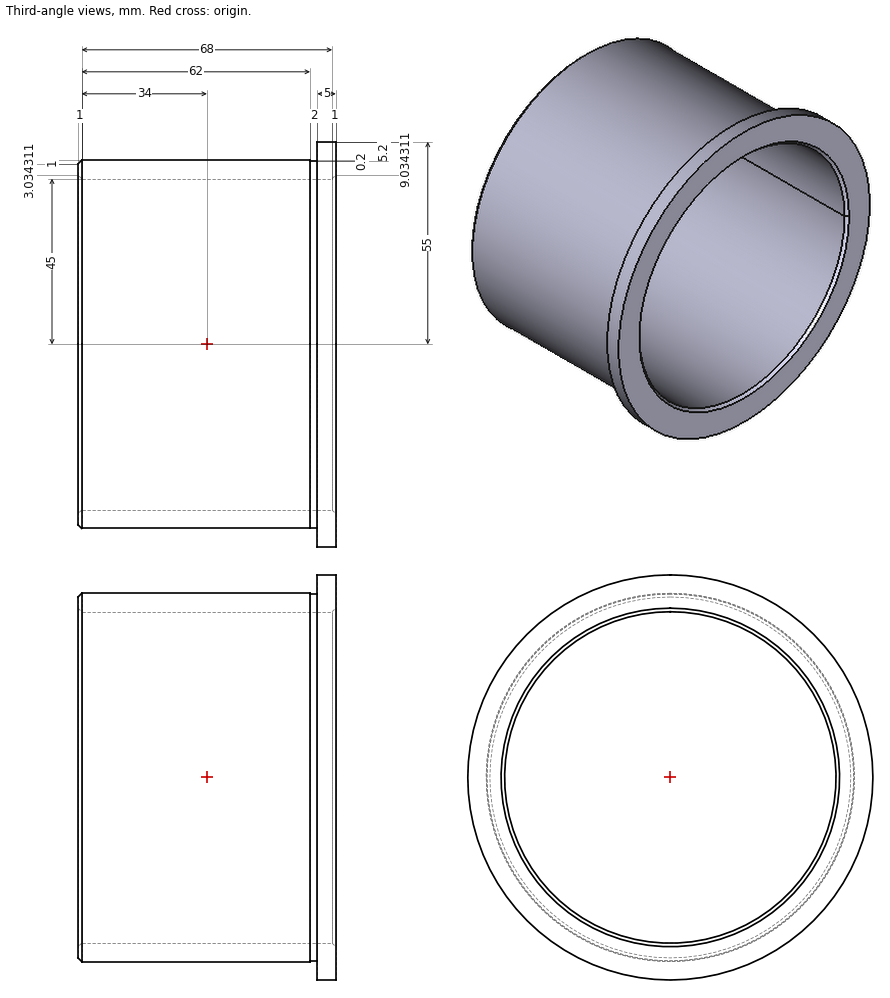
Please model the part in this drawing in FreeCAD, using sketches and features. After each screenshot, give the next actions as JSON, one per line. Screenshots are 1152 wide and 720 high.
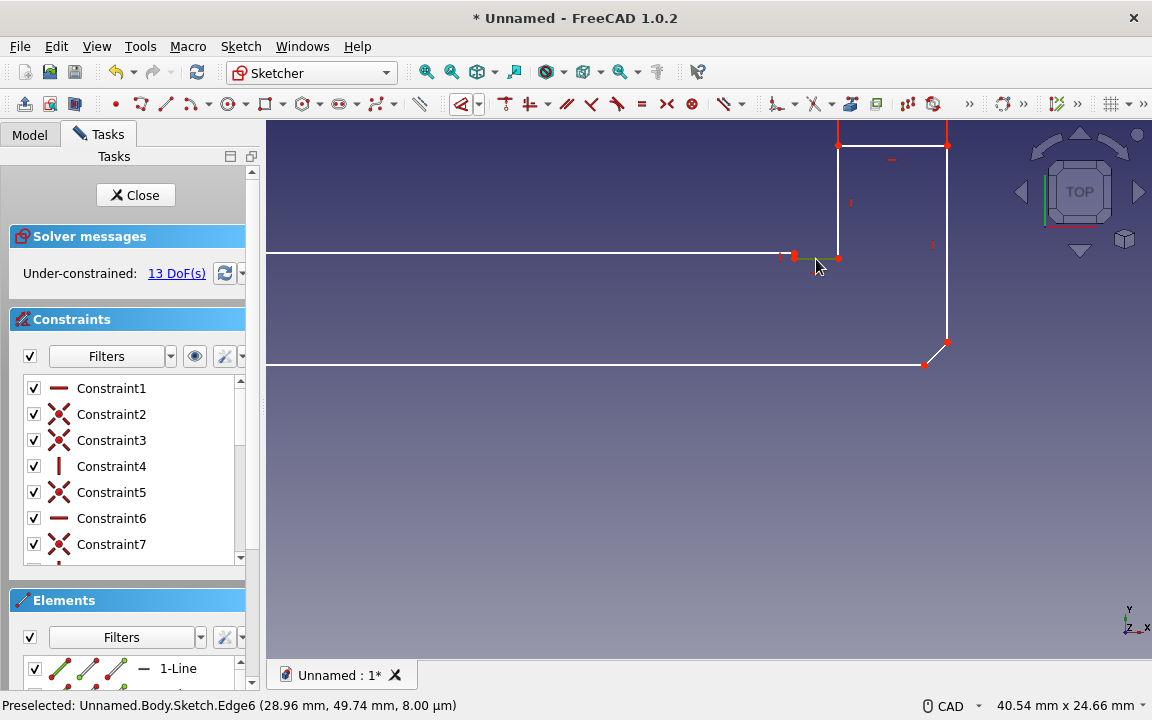
{"action": "key", "text": "l"}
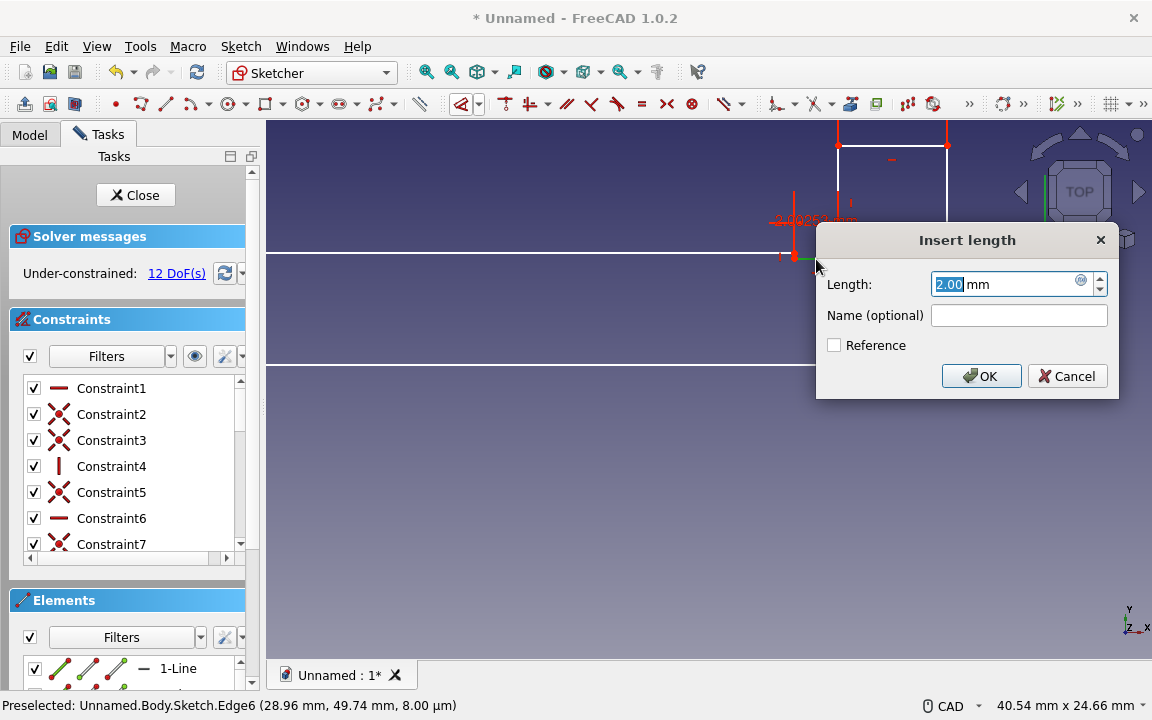
{"action": "type", "text": "2"}
{"action": "key", "text": "Return"}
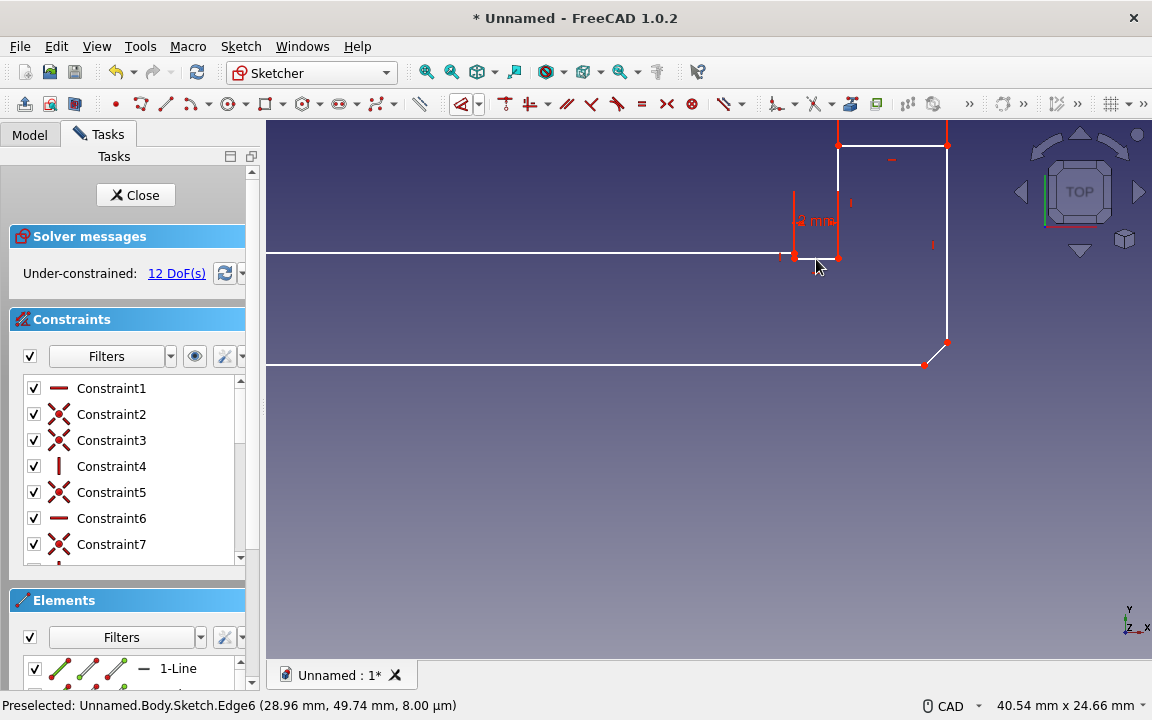
{"action": "left_click", "coordinate": [480, 365]}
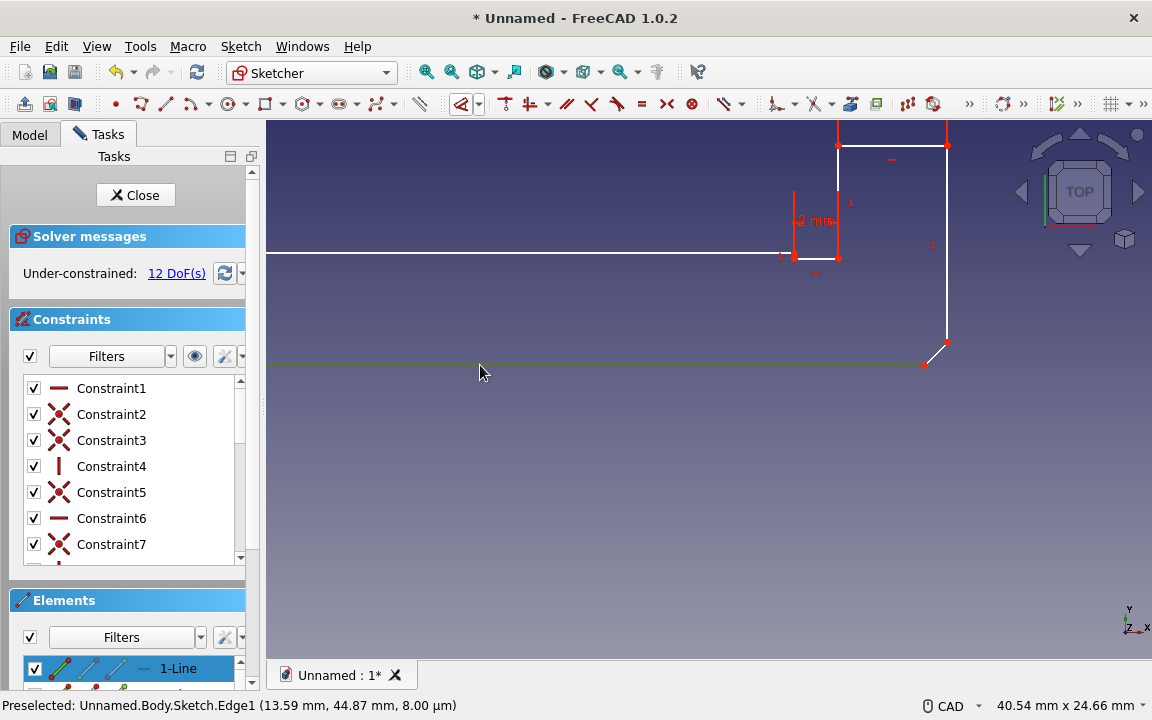
{"action": "key", "text": "l"}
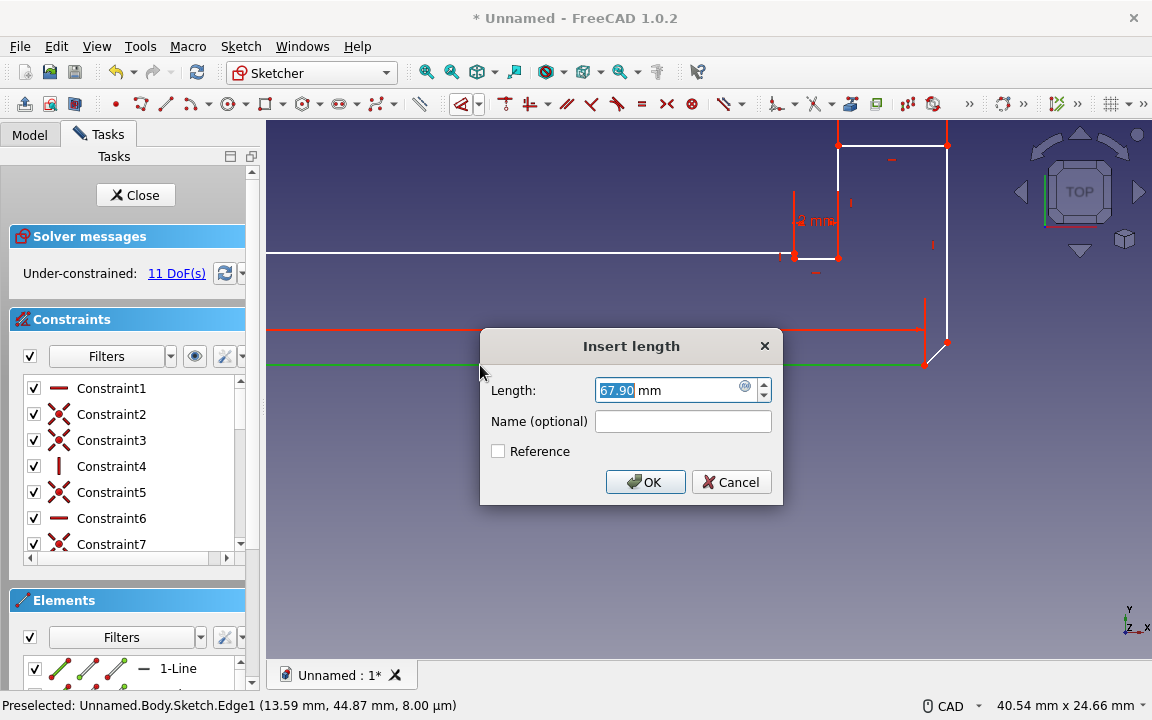
{"action": "type", "text": "68"}
{"action": "key", "text": "Return"}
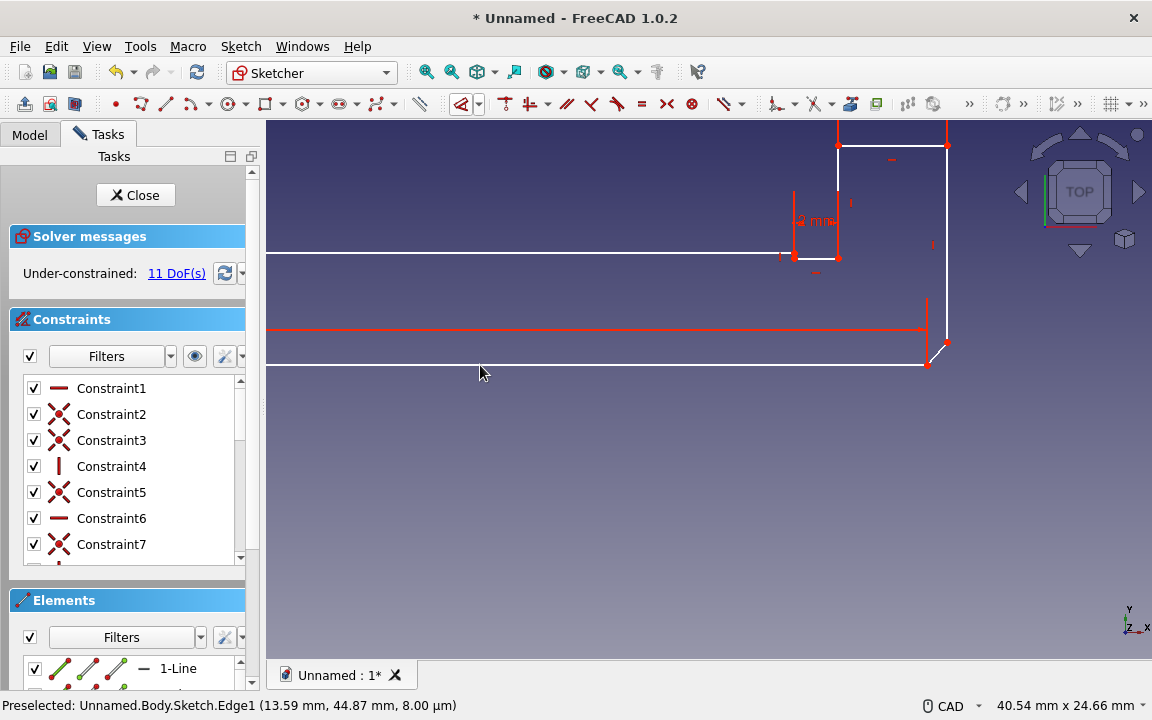
{"action": "left_click", "coordinate": [388, 253]}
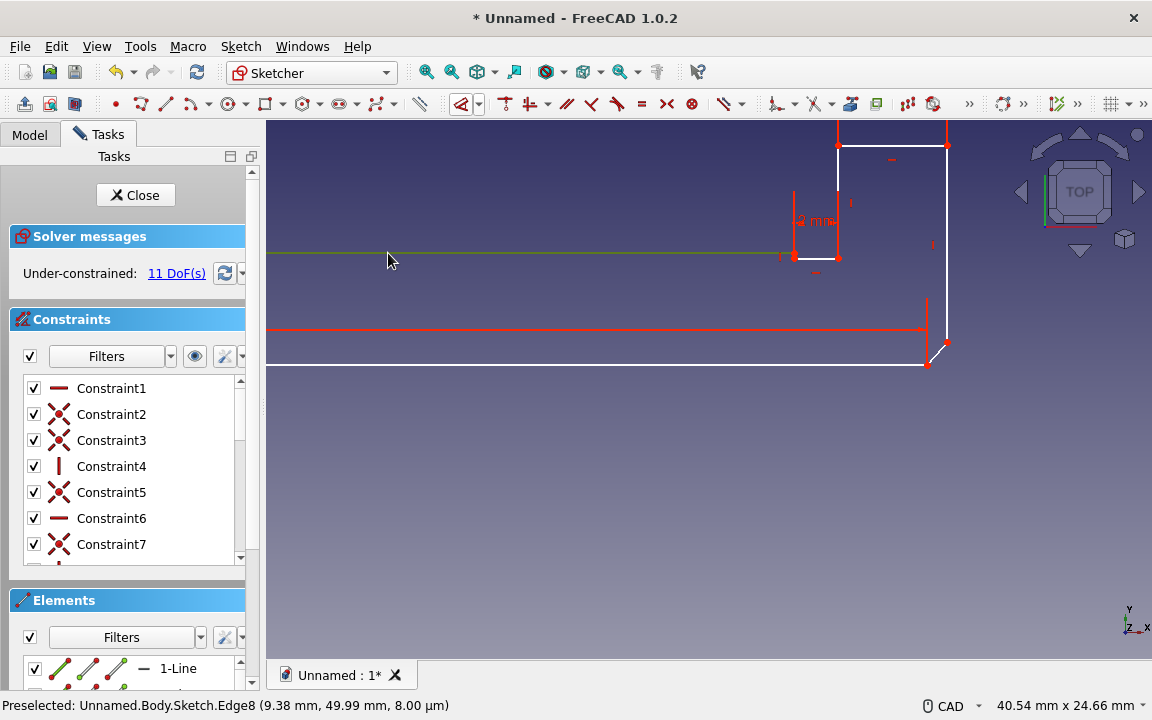
{"action": "left_click", "coordinate": [478, 104]}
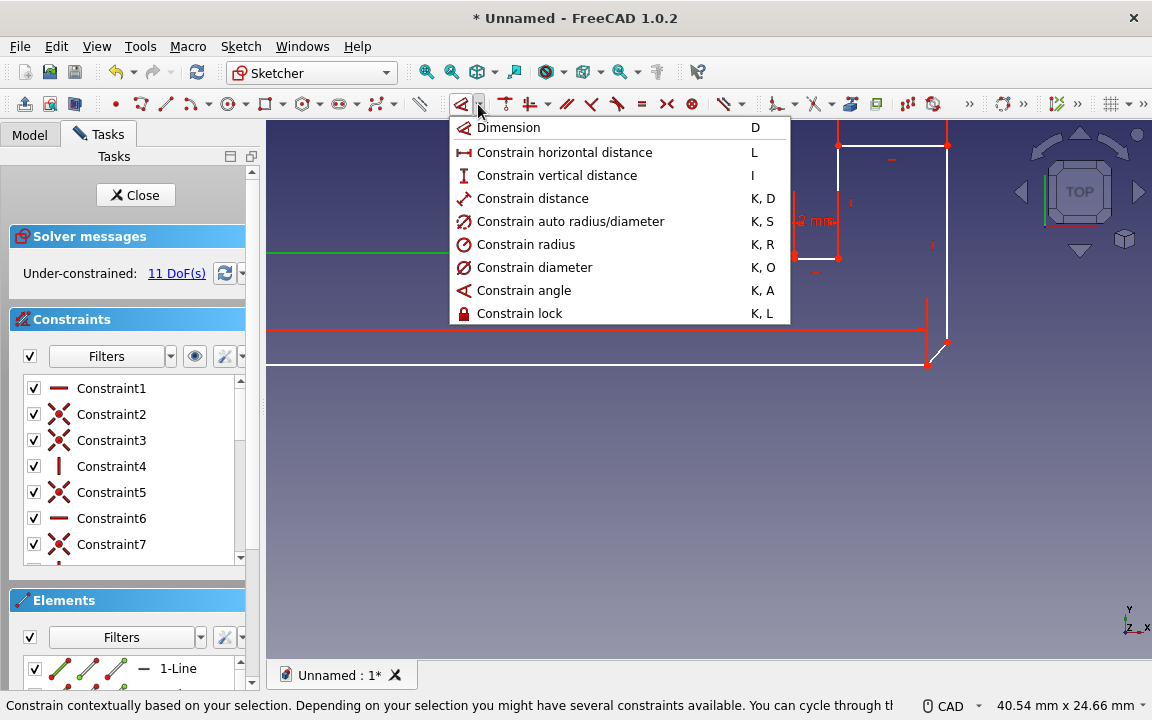
{"action": "left_click", "coordinate": [620, 152]}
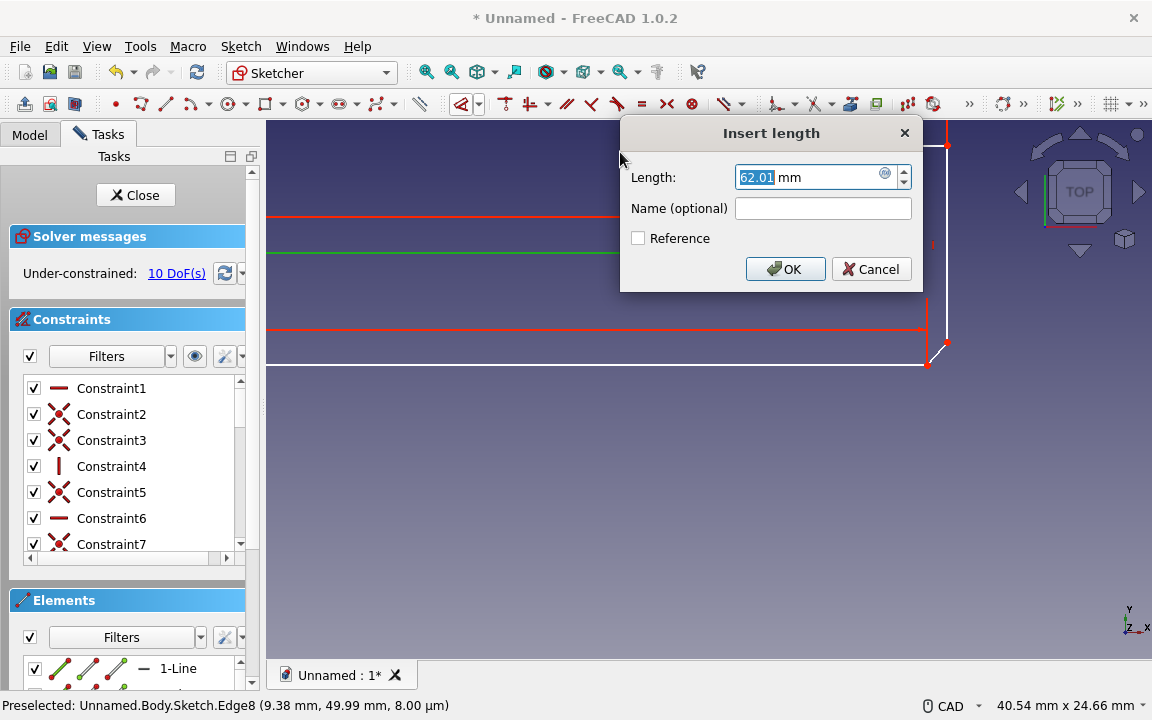
{"action": "type", "text": "62"}
{"action": "key", "text": "Return"}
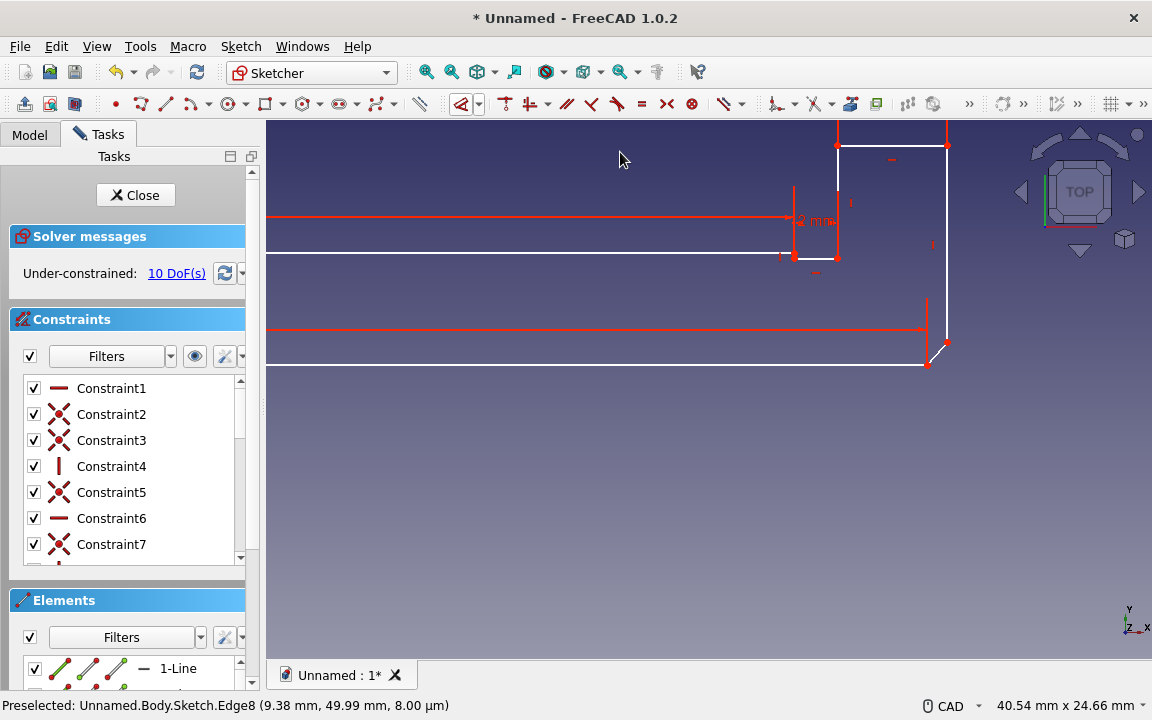
{"action": "scroll", "coordinate": [933, 359], "scroll_direction": "up", "scroll_amount": 3}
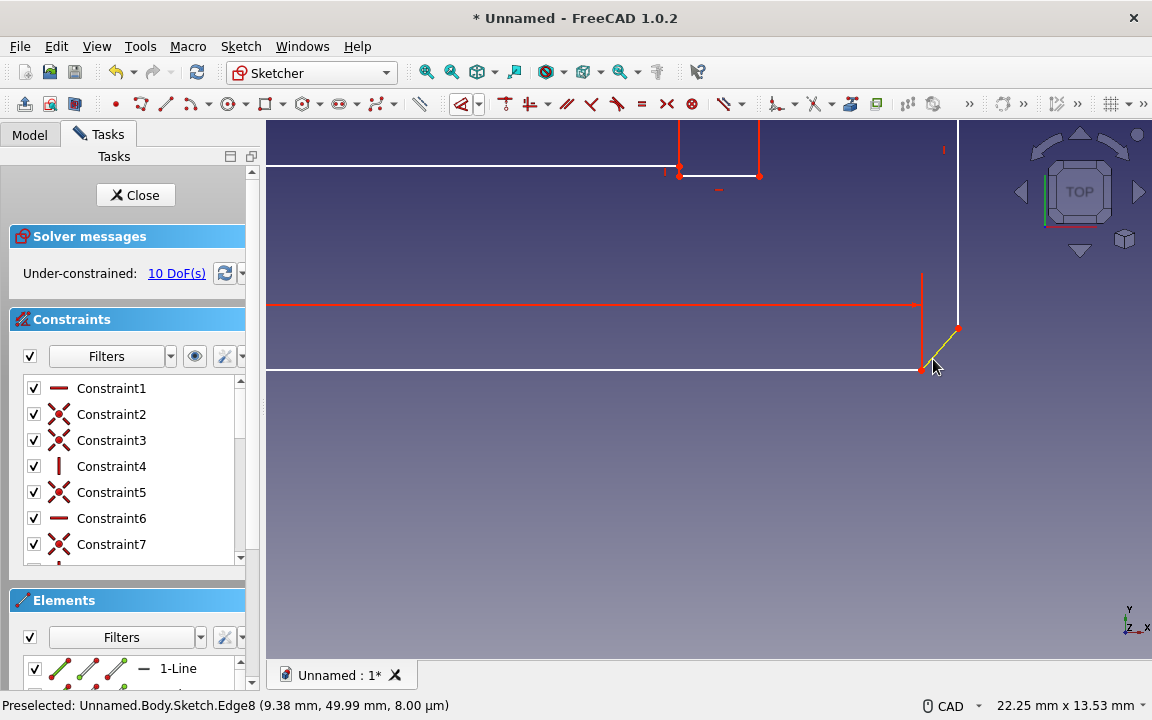
{"action": "left_click", "coordinate": [933, 358]}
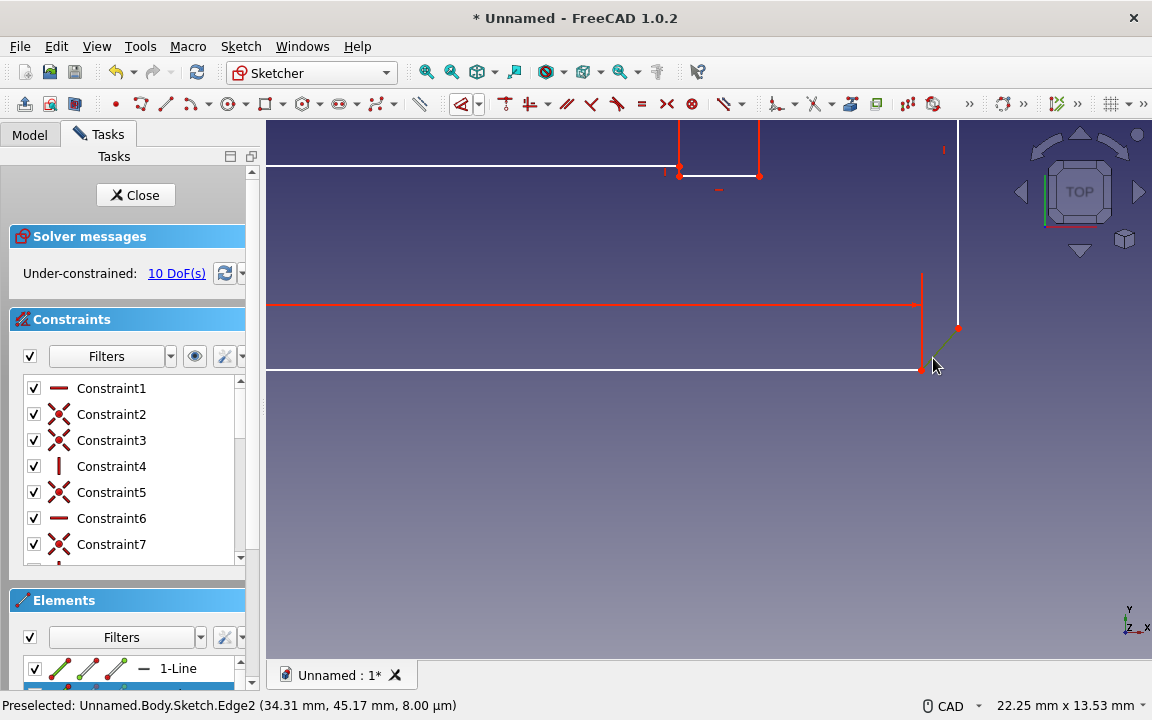
{"action": "key", "text": "l"}